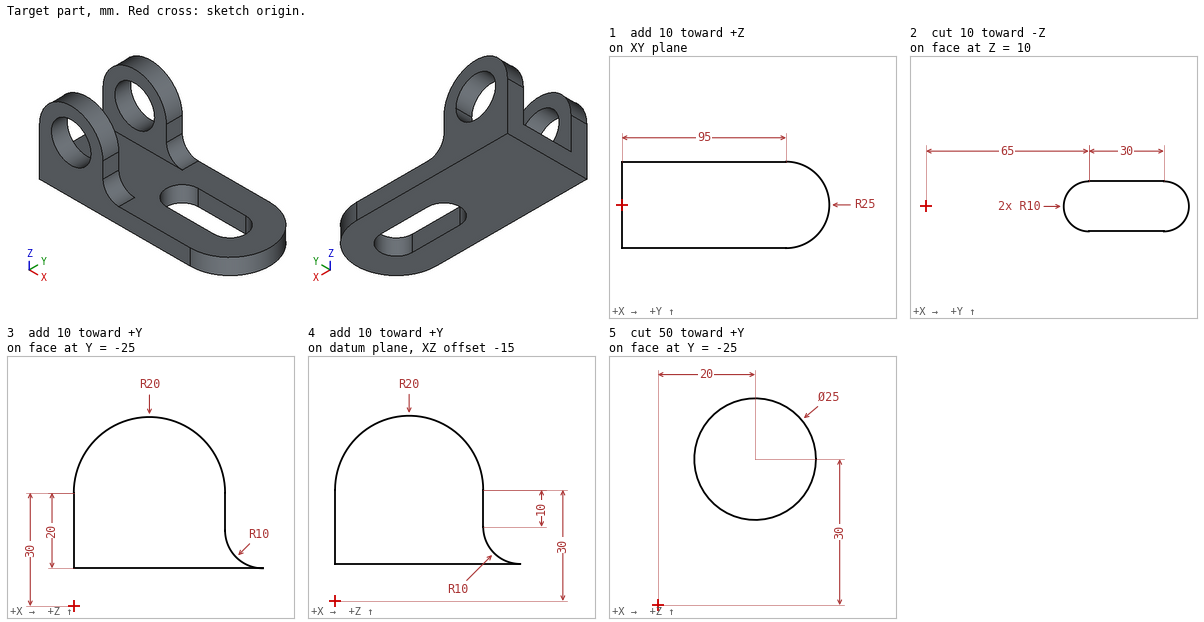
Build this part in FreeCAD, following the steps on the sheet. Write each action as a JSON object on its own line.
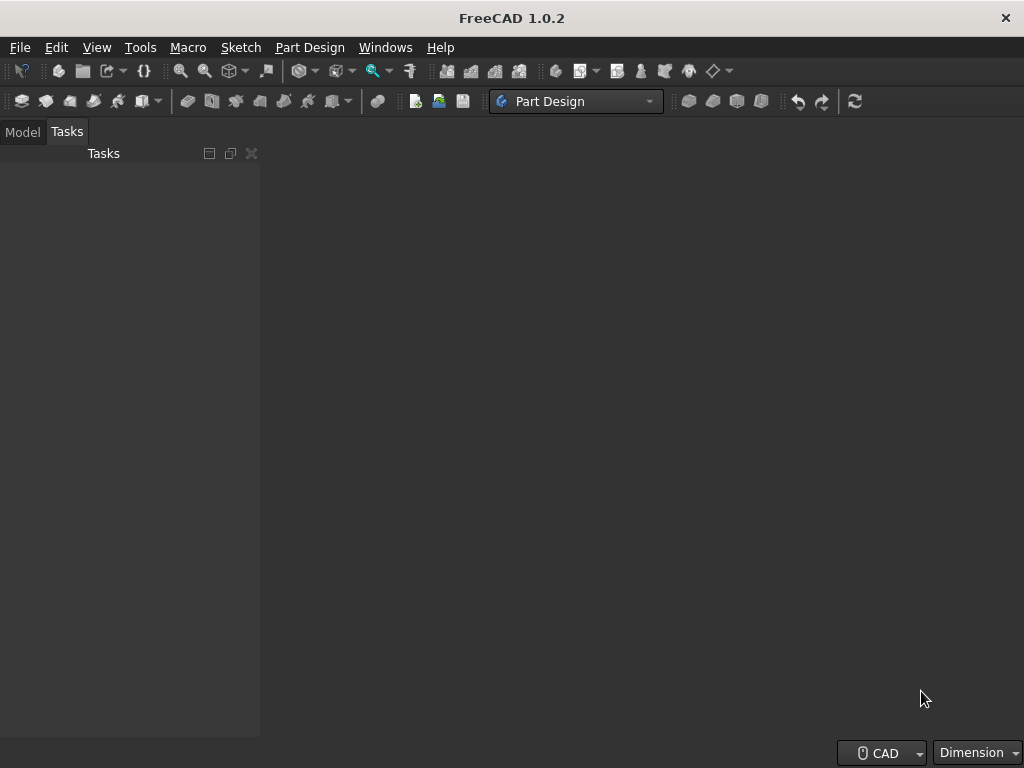
{"action": "left_click", "coordinate": [416, 102]}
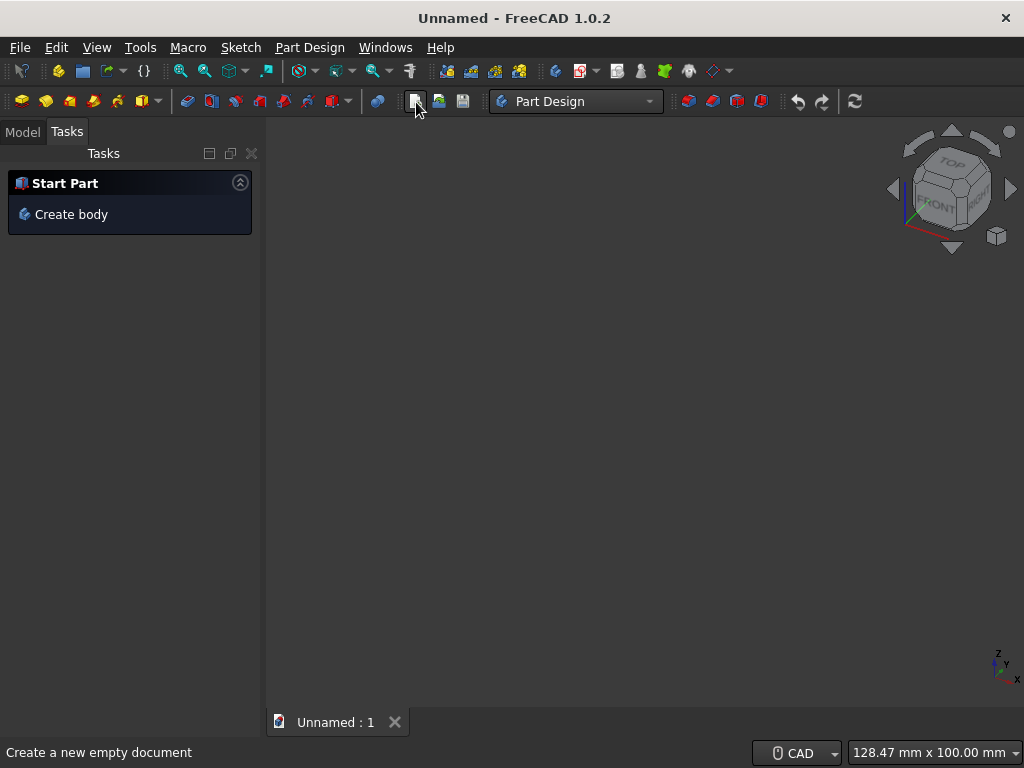
{"action": "left_click", "coordinate": [580, 72]}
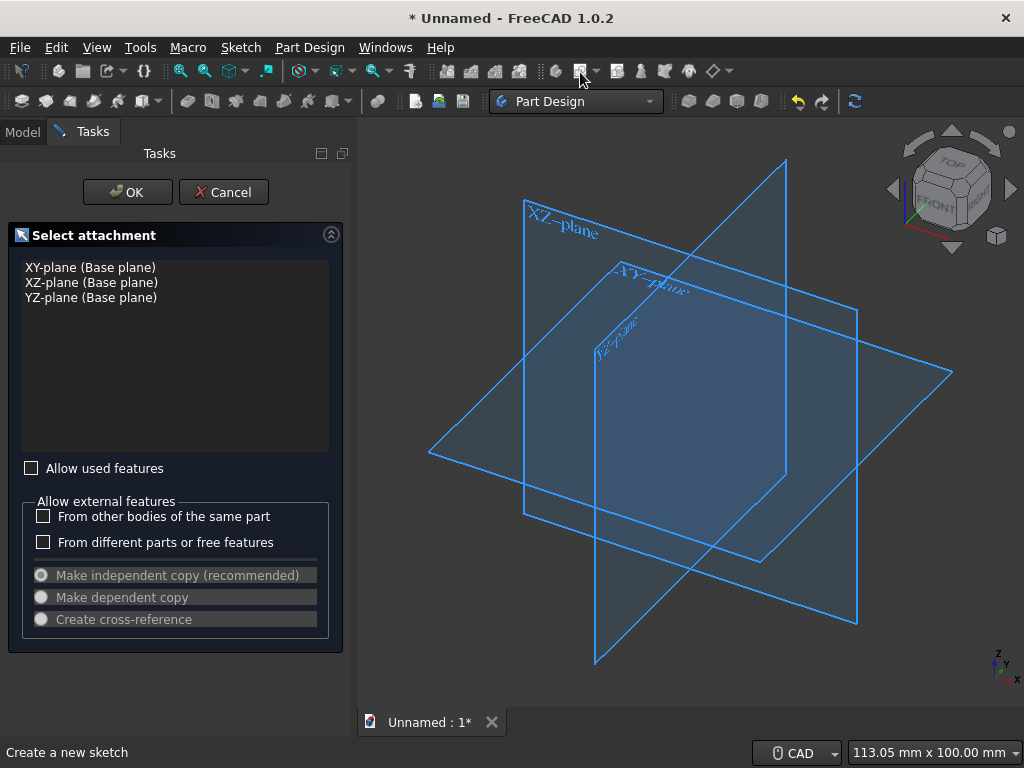
{"action": "left_click", "coordinate": [82, 268]}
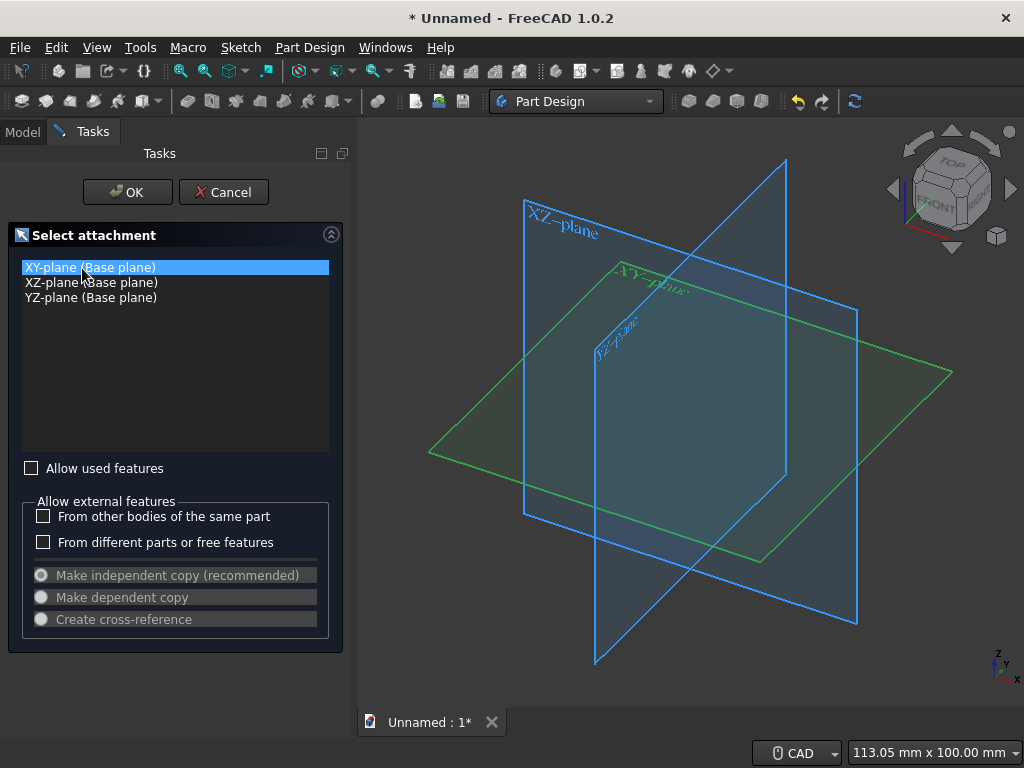
{"action": "left_click", "coordinate": [128, 192]}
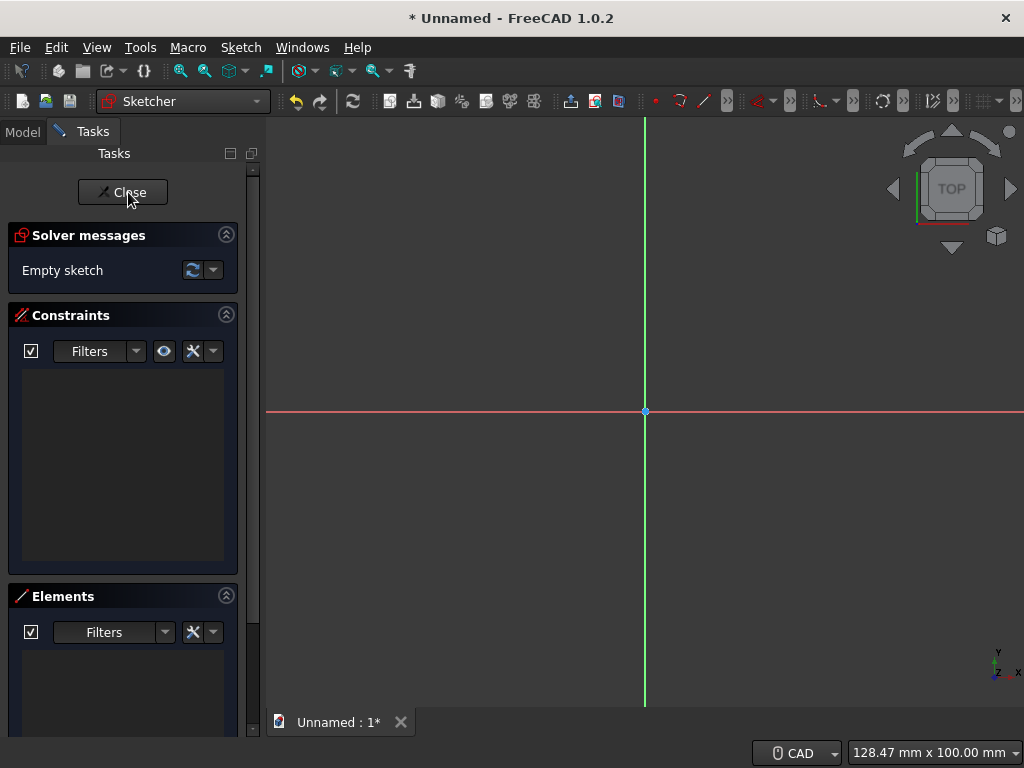
{"action": "scroll", "coordinate": [294, 412], "scroll_direction": "down", "scroll_amount": 4}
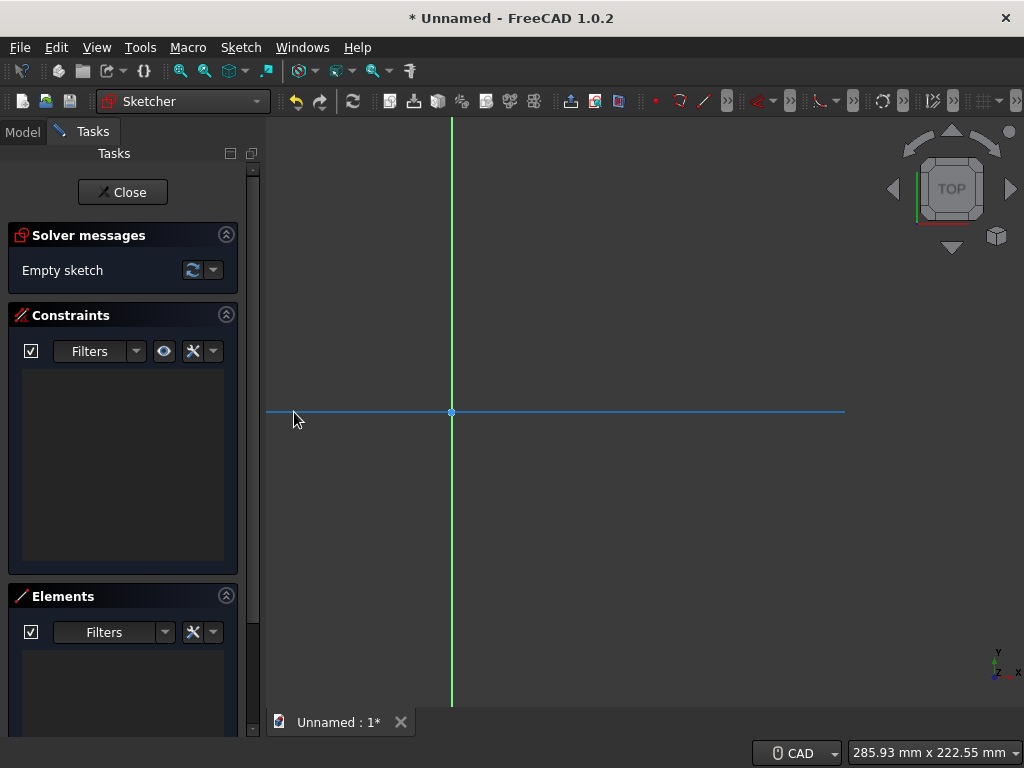
{"action": "left_click", "coordinate": [680, 102]}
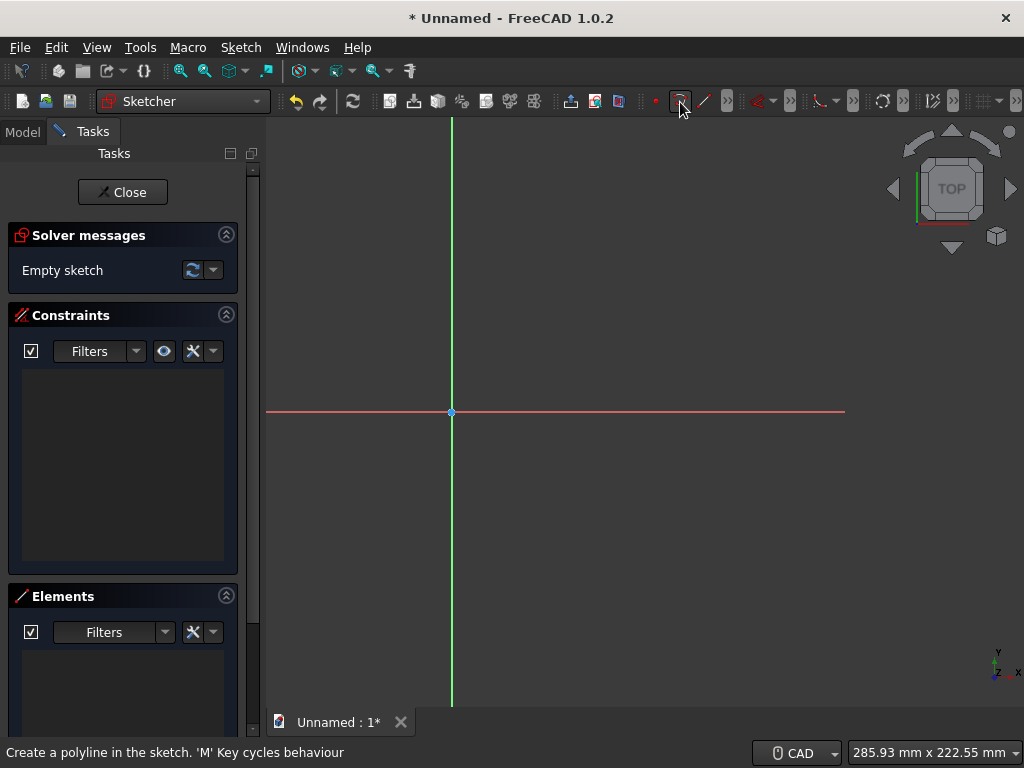
{"action": "left_click", "coordinate": [704, 346]}
{"action": "left_click", "coordinate": [452, 346]}
{"action": "left_click", "coordinate": [461, 479]}
{"action": "left_click", "coordinate": [704, 479]}
{"action": "right_click", "coordinate": [704, 479]}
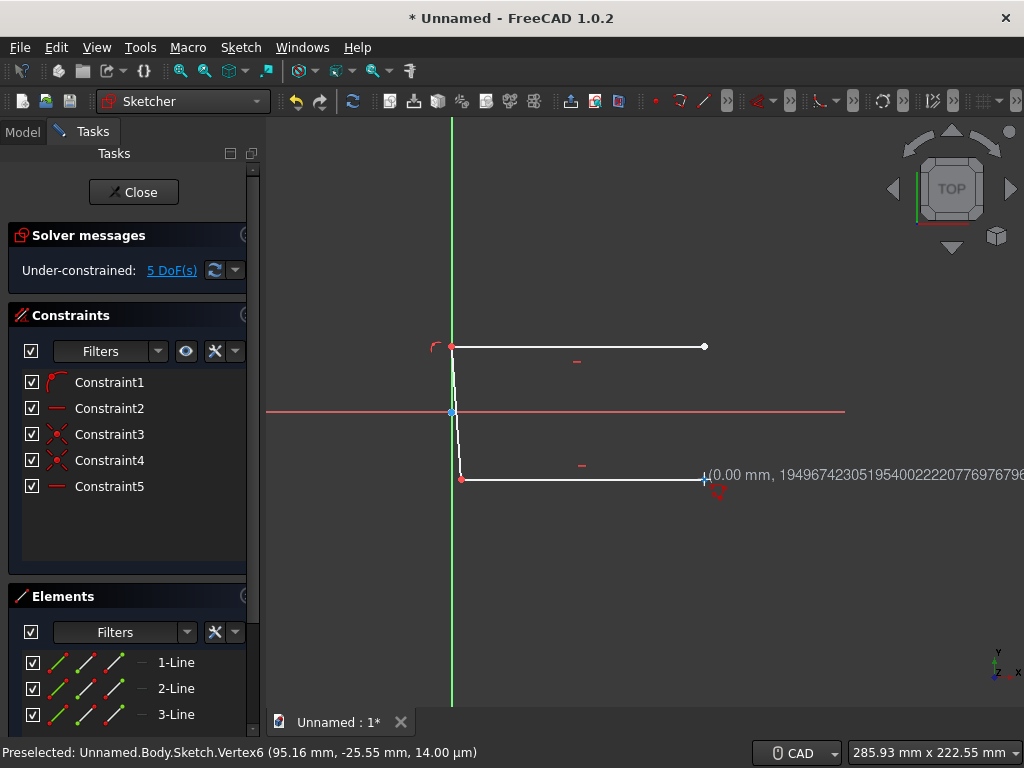
{"action": "key", "text": "g 3 a"}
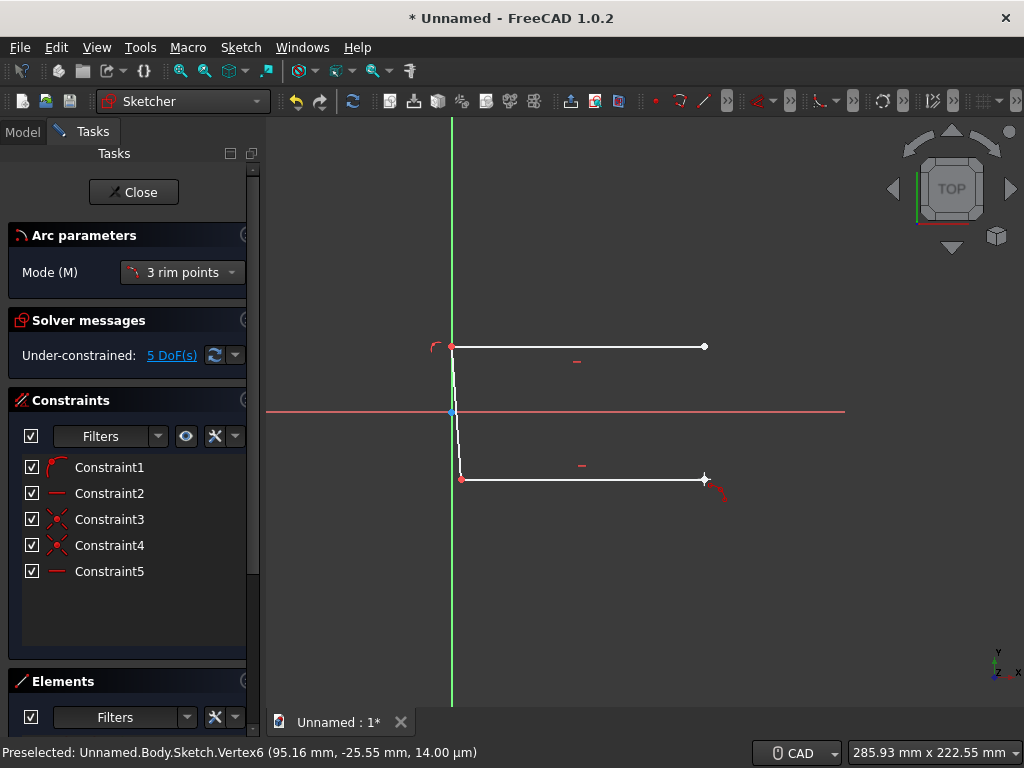
{"action": "left_click", "coordinate": [704, 480]}
{"action": "left_click", "coordinate": [704, 347]}
{"action": "left_click", "coordinate": [767, 433]}
{"action": "key", "text": "Escape"}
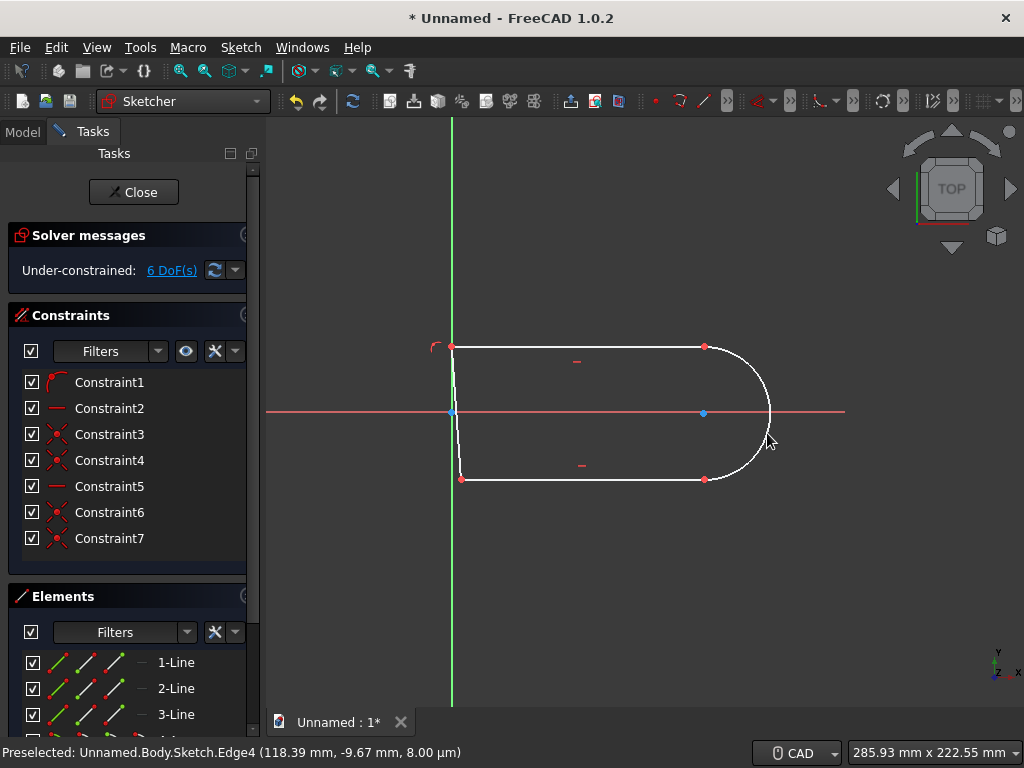
{"action": "left_click", "coordinate": [628, 347]}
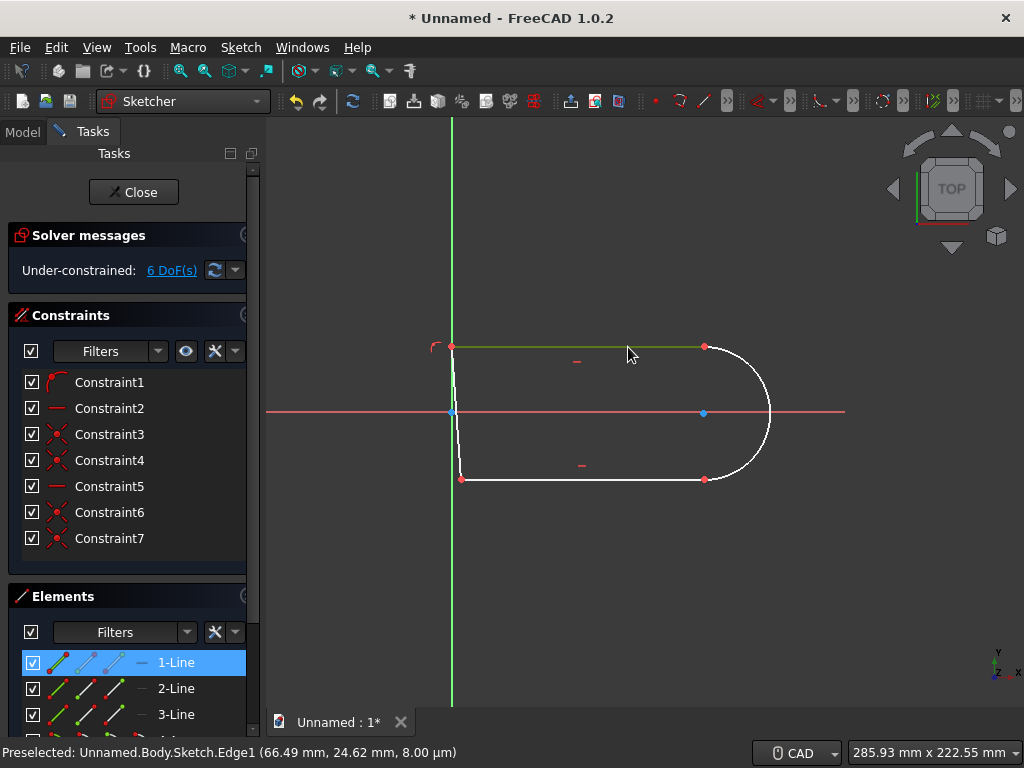
{"action": "left_click", "coordinate": [758, 453]}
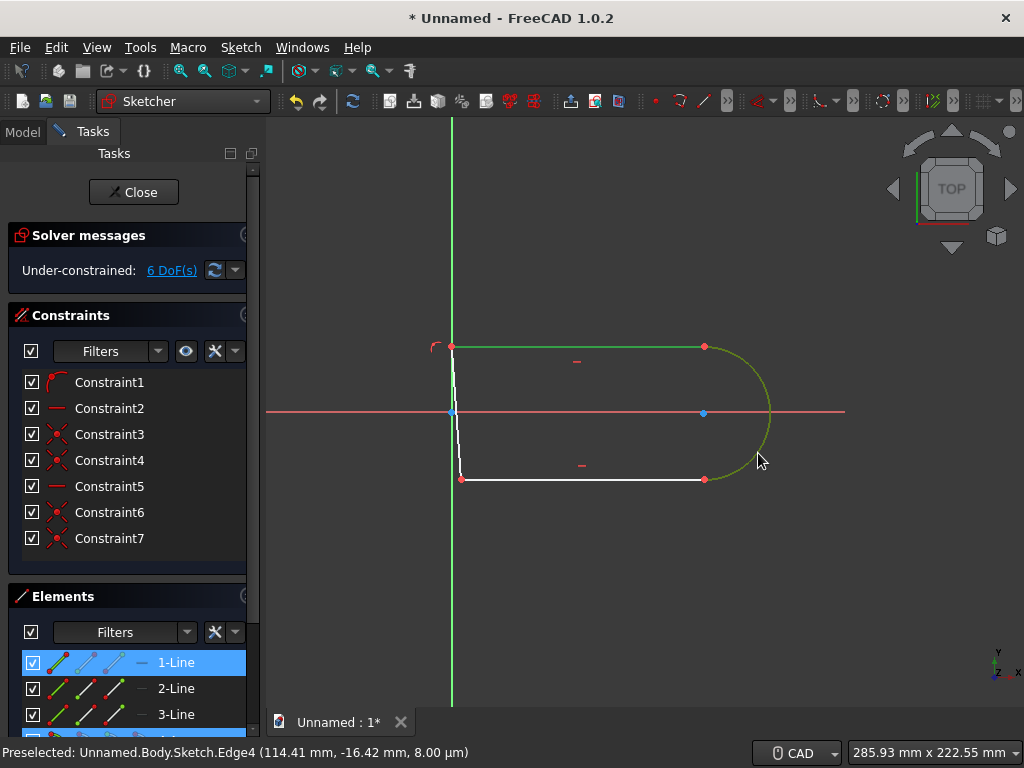
{"action": "key", "text": "t"}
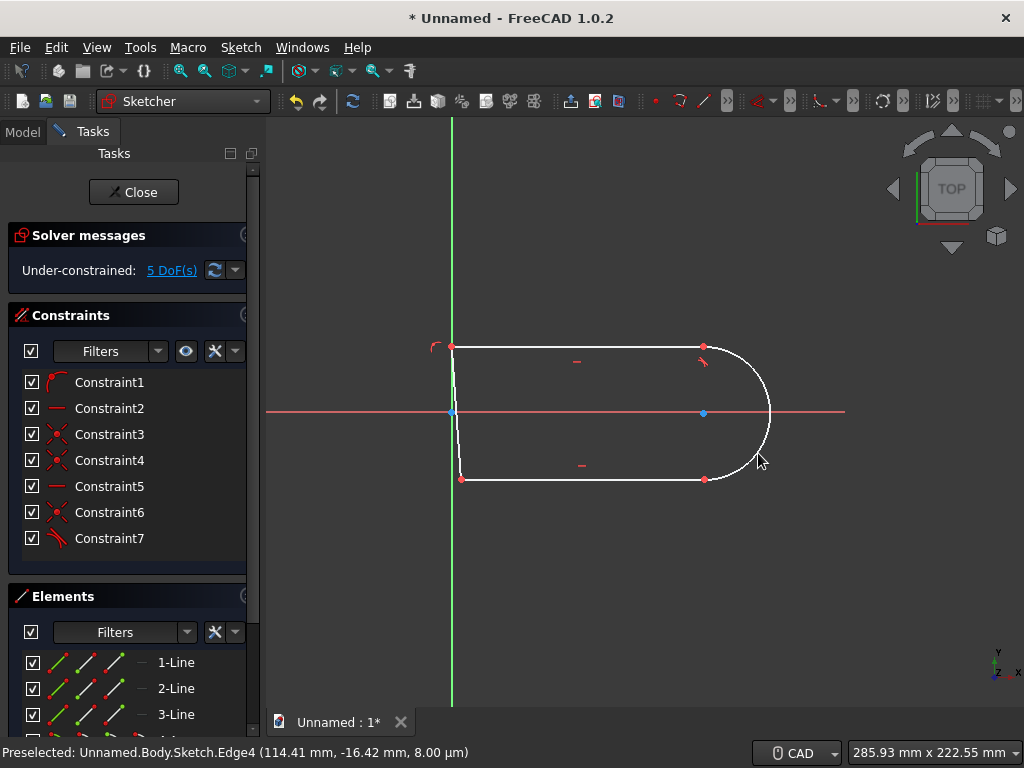
{"action": "left_click", "coordinate": [534, 480]}